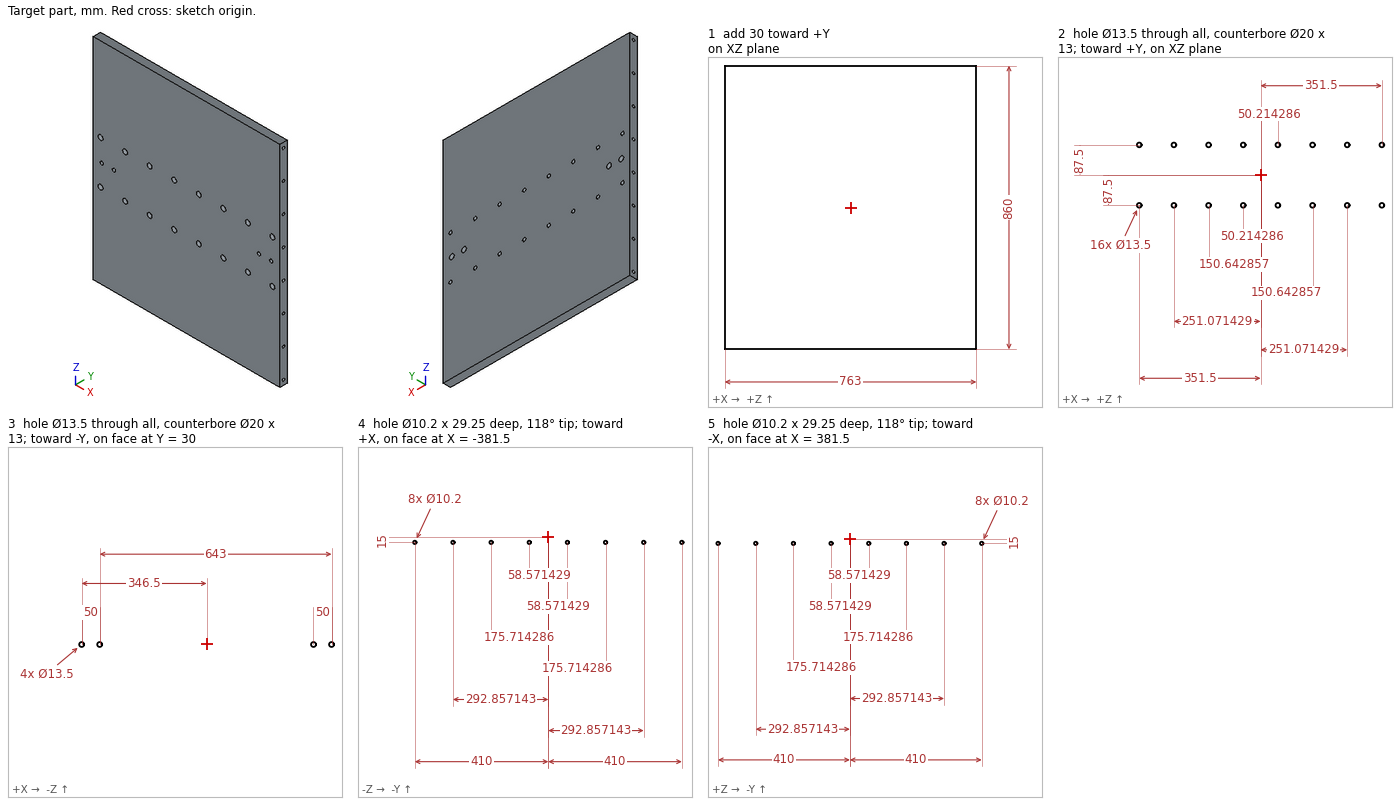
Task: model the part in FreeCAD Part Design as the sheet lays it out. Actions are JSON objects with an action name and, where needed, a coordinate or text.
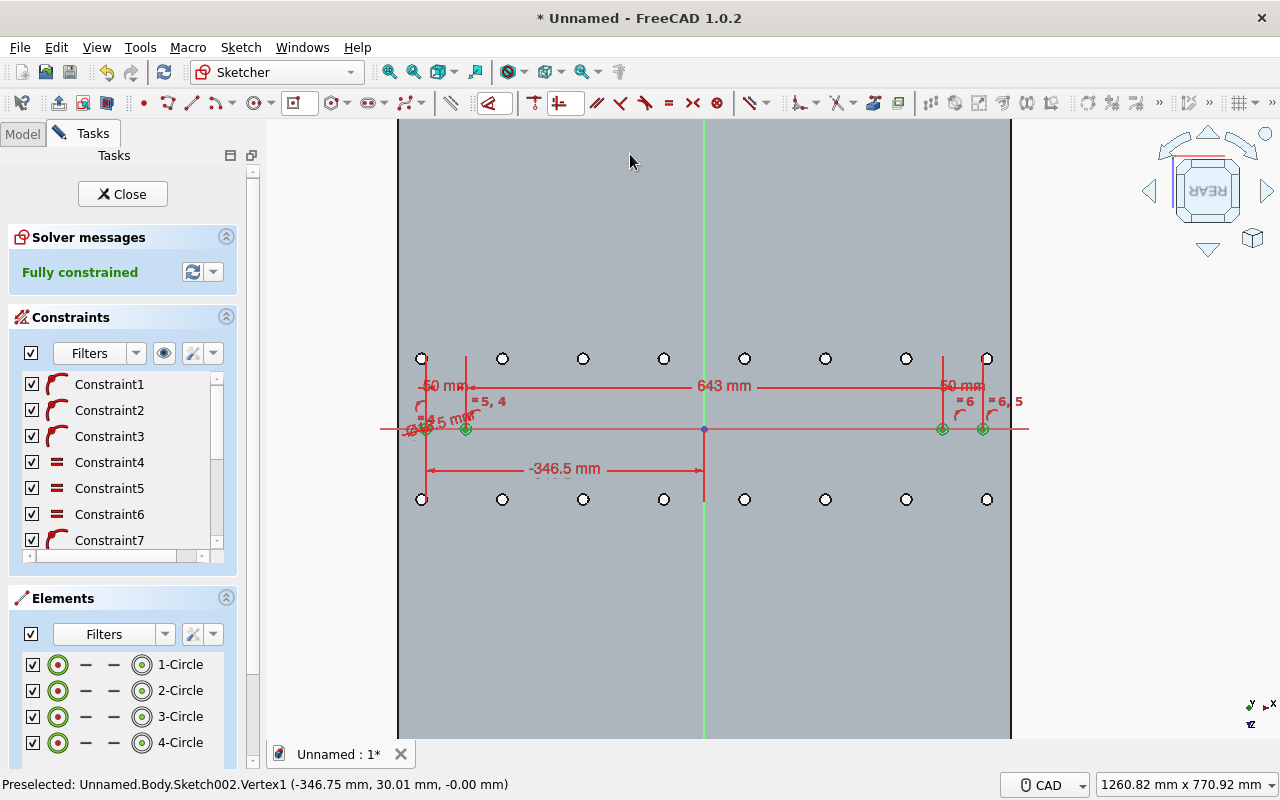
{"action": "left_click", "coordinate": [123, 194]}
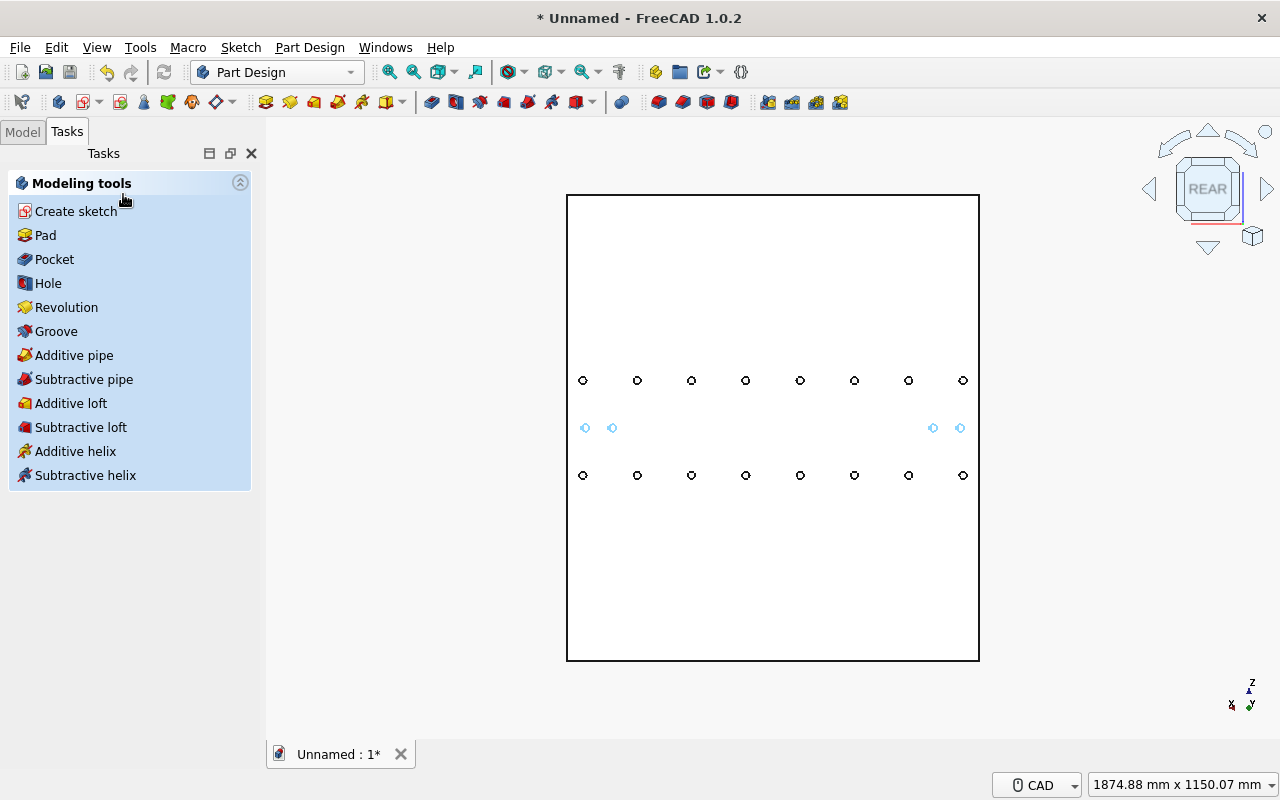
{"action": "left_click", "coordinate": [456, 102]}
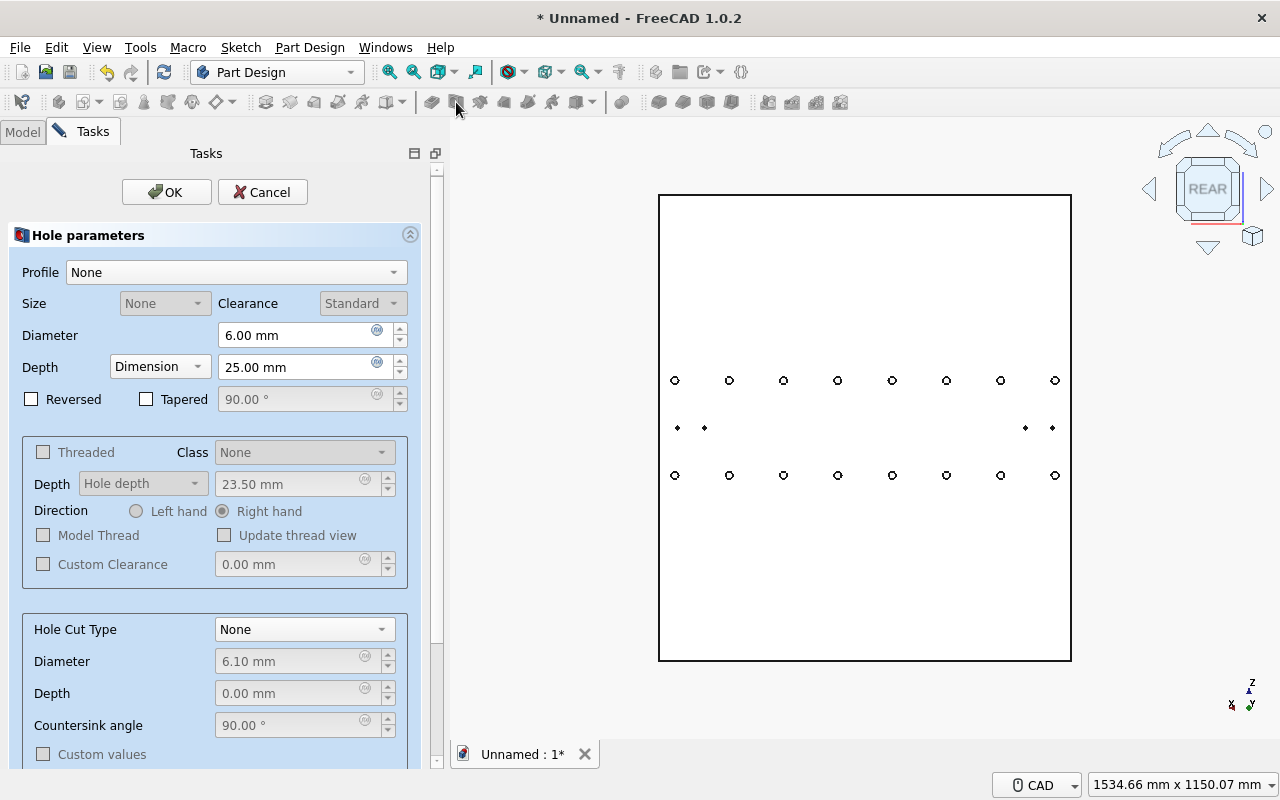
{"action": "triple_click", "coordinate": [305, 335]}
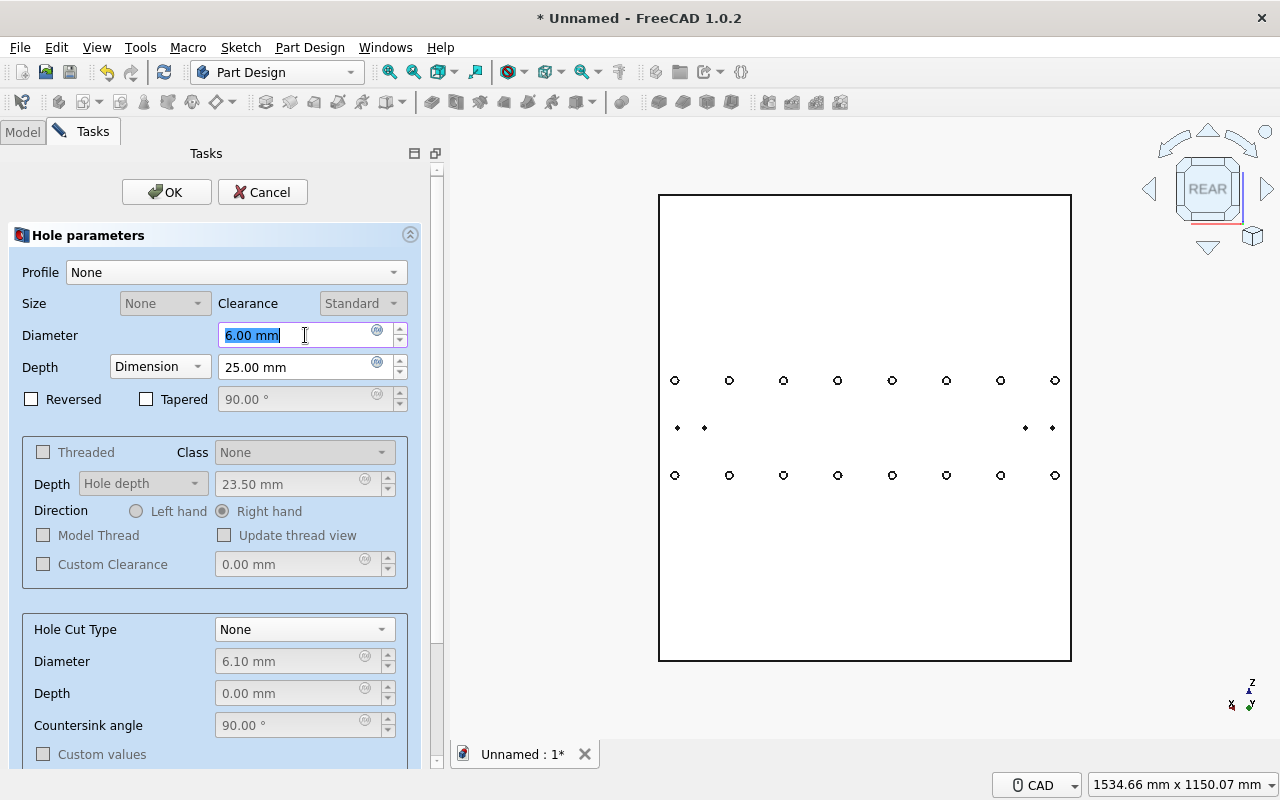
{"action": "type", "text": "13.5"}
{"action": "key", "text": "Tab"}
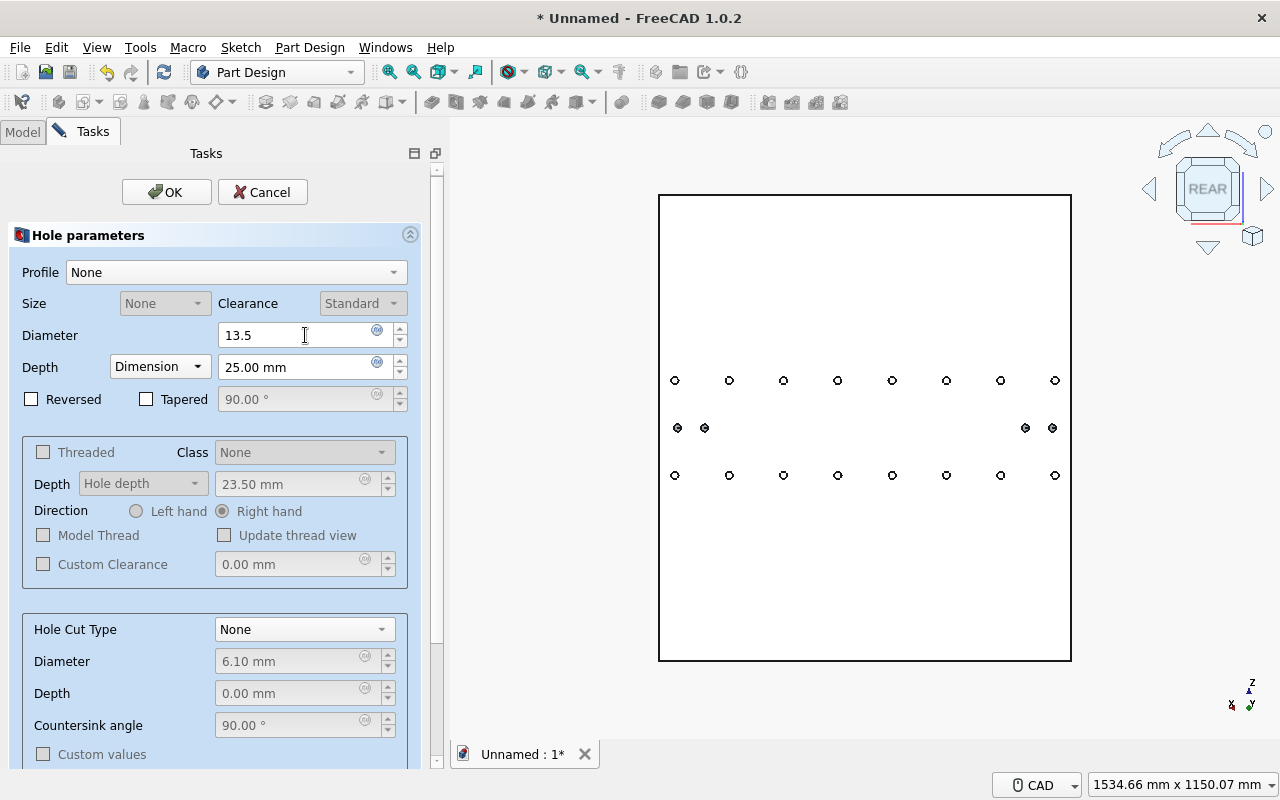
{"action": "left_click", "coordinate": [161, 366]}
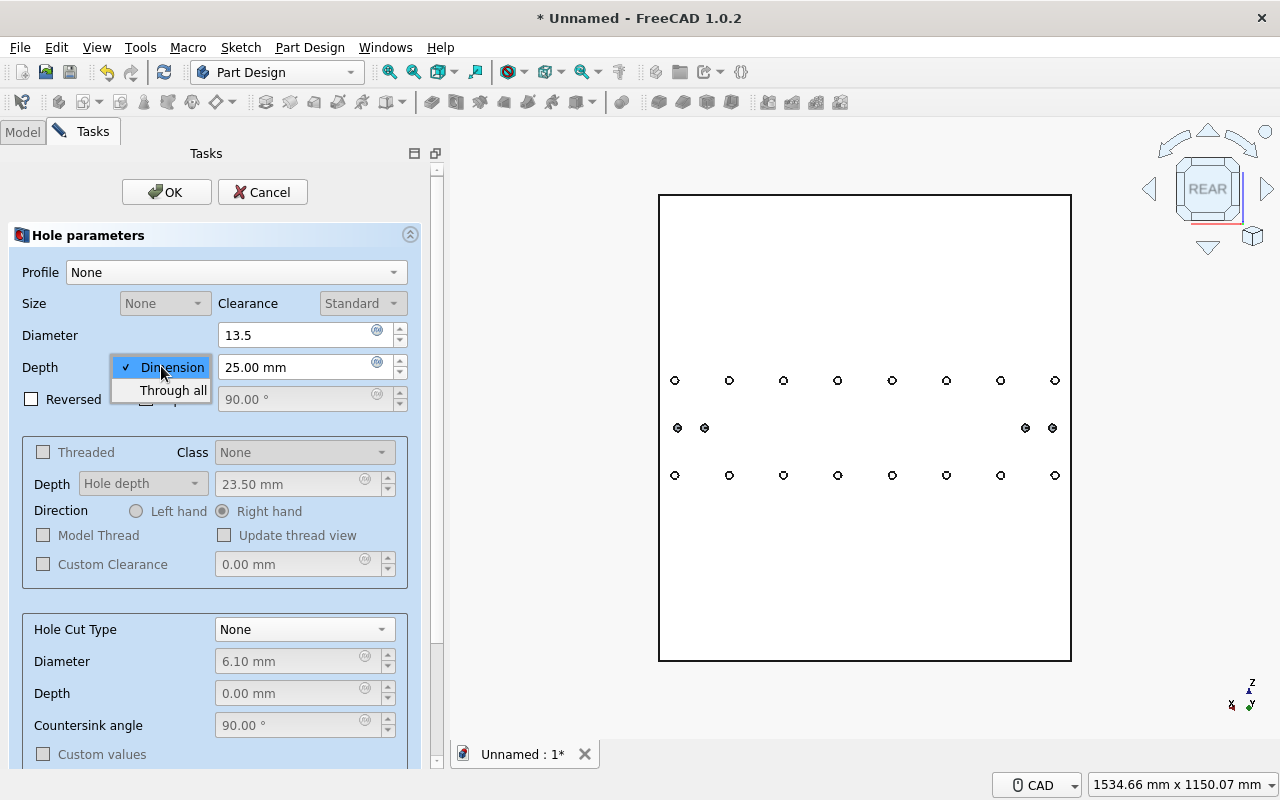
{"action": "left_click", "coordinate": [160, 390]}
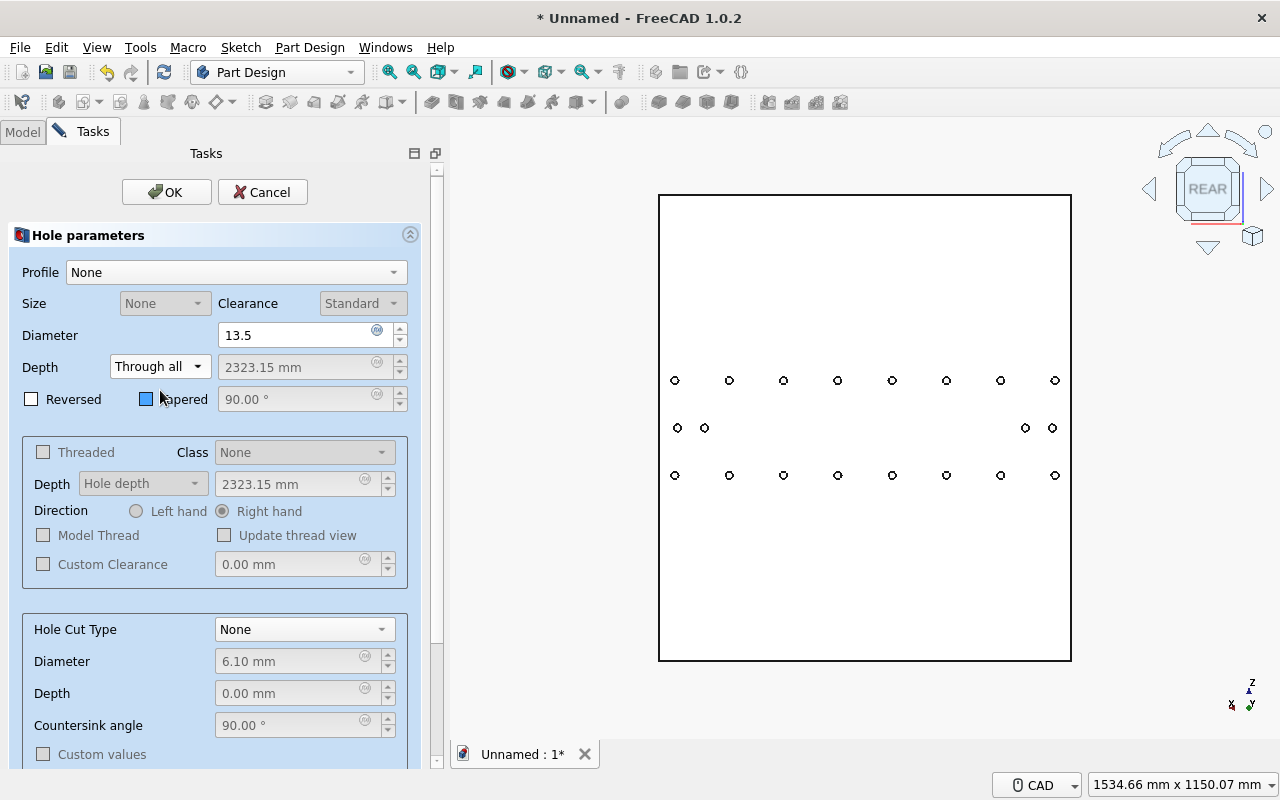
{"action": "left_click", "coordinate": [306, 630]}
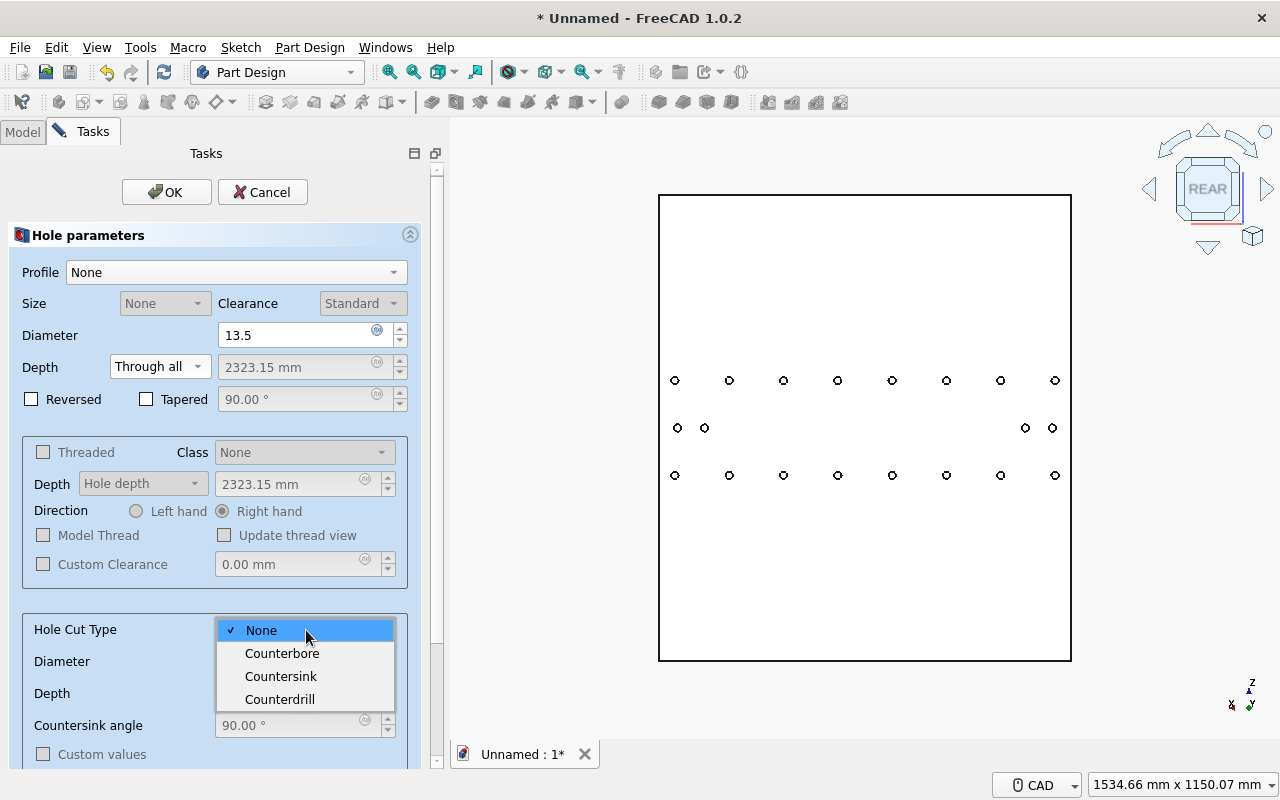
{"action": "left_click", "coordinate": [304, 654]}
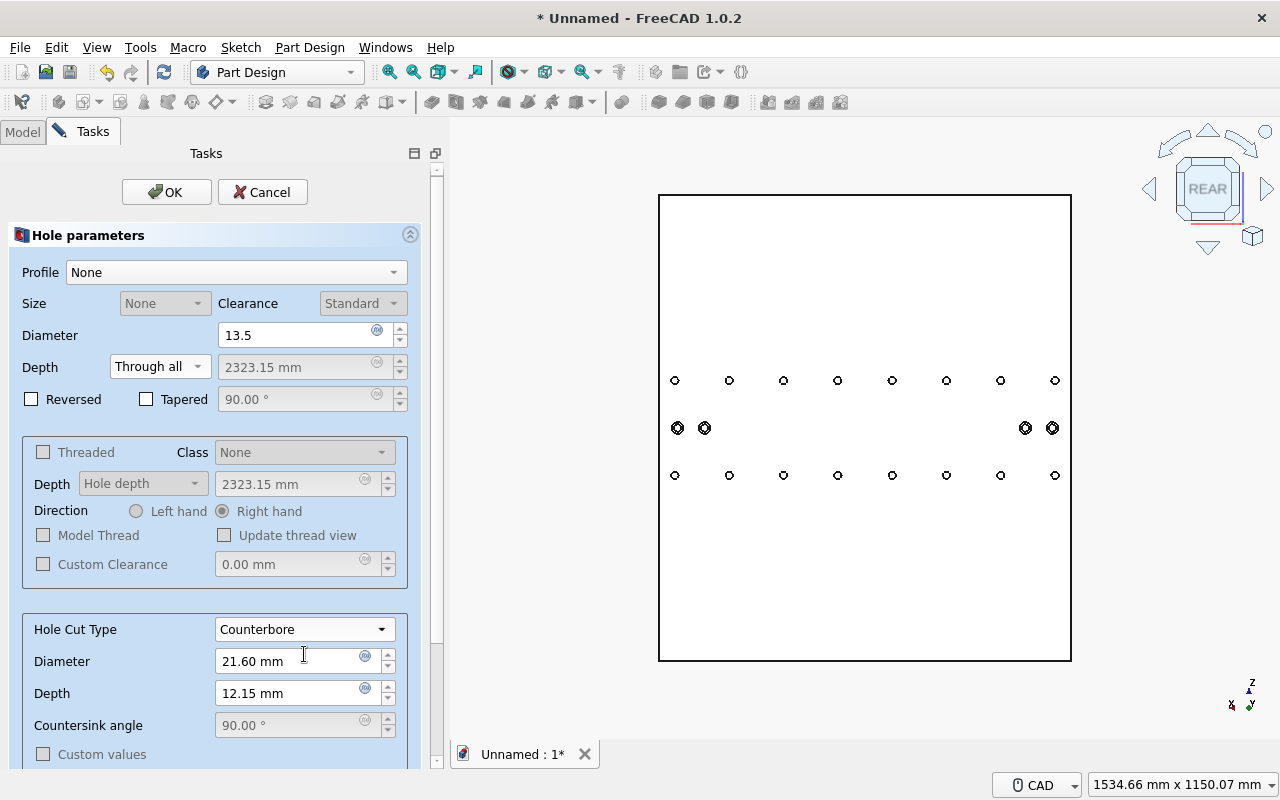
{"action": "triple_click", "coordinate": [298, 661]}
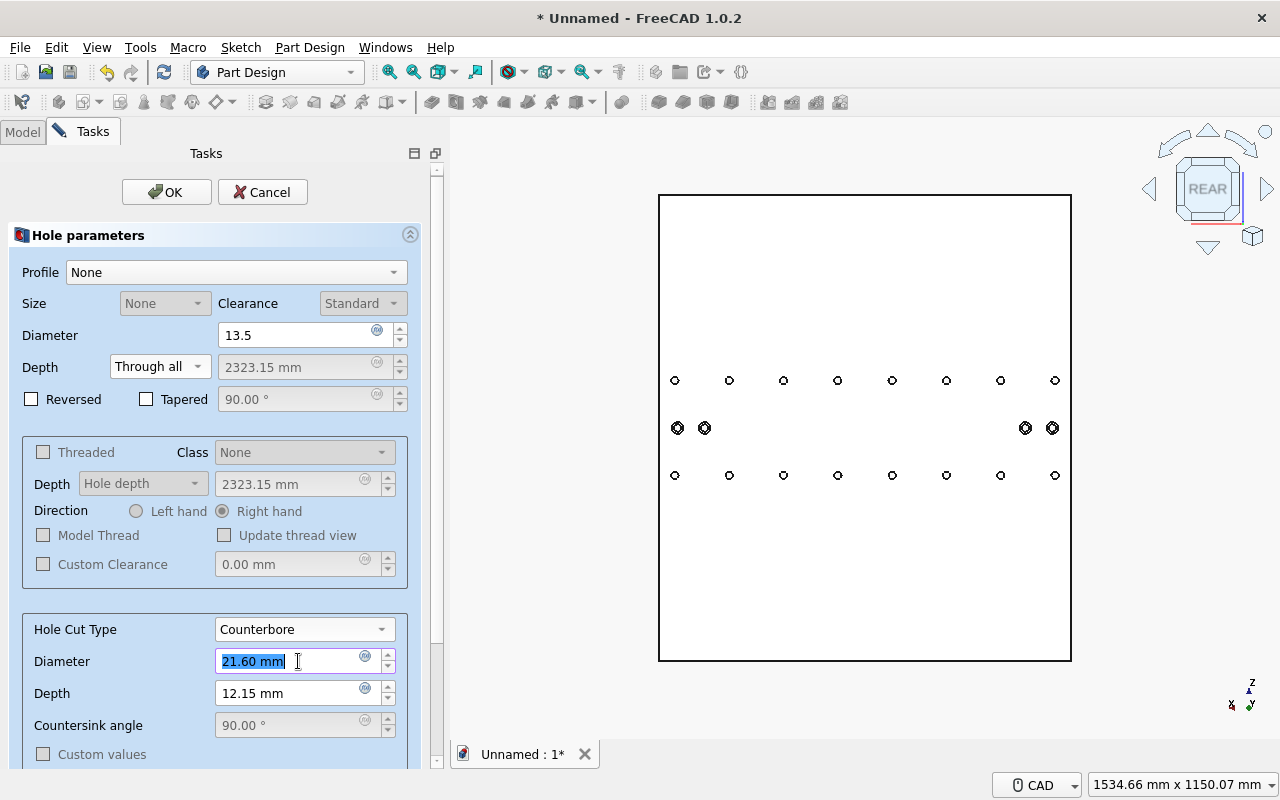
{"action": "type", "text": "20"}
{"action": "key", "text": "Tab"}